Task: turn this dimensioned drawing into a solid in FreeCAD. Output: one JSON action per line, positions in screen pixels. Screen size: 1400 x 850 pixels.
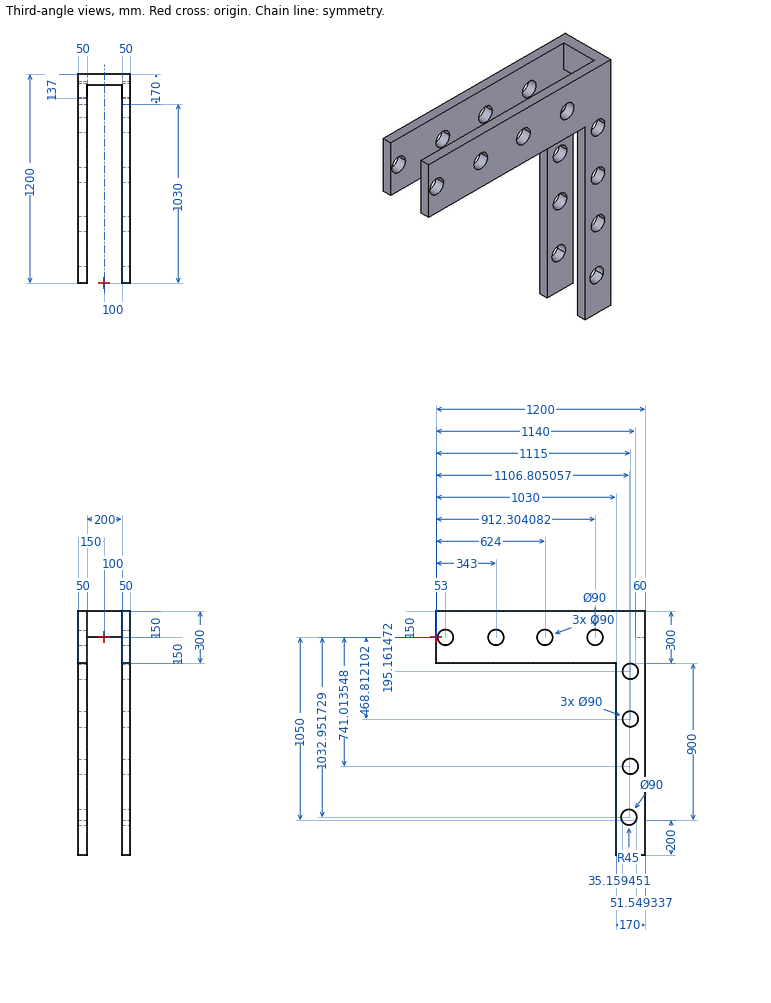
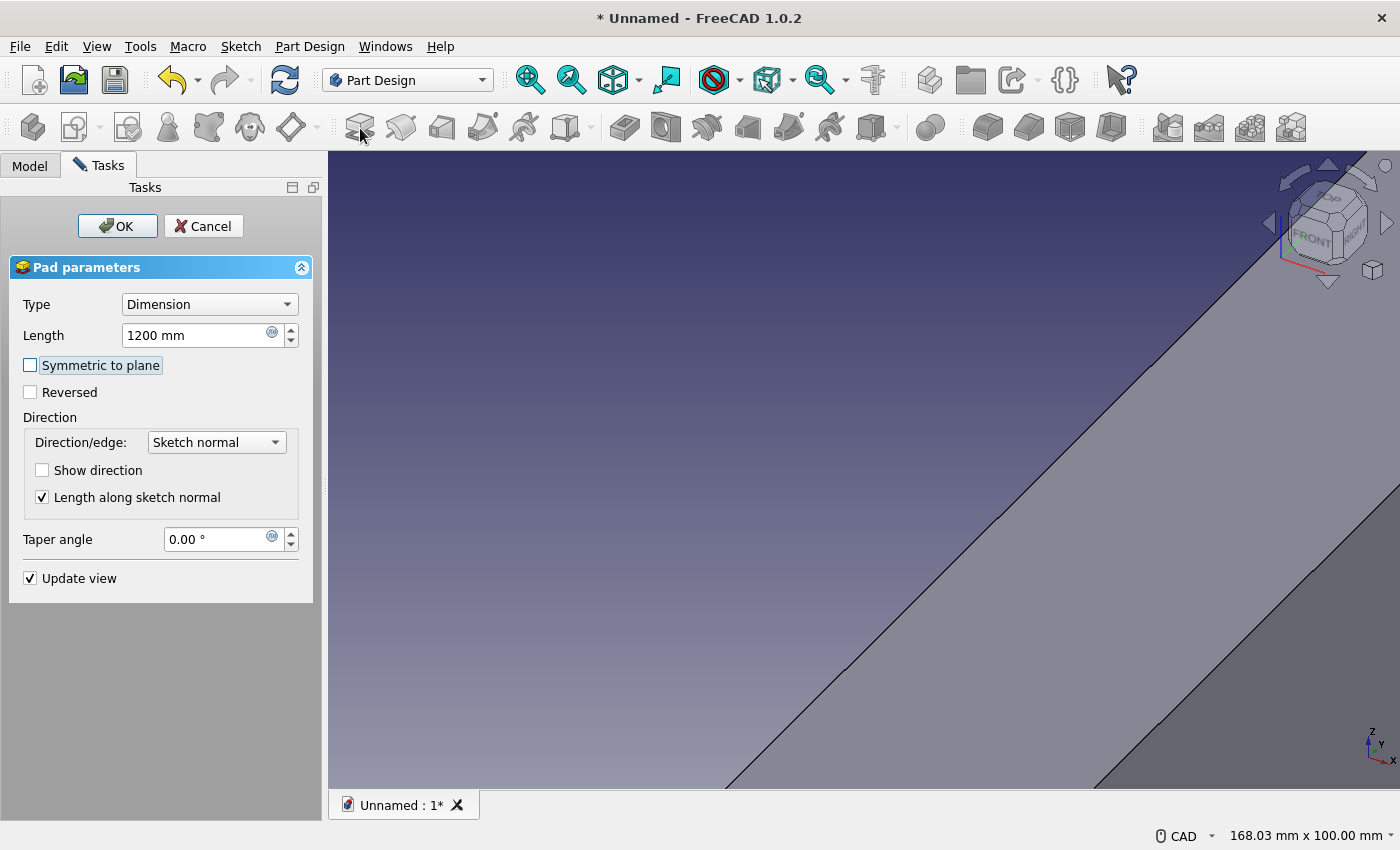
{"action": "left_click", "coordinate": [31, 392]}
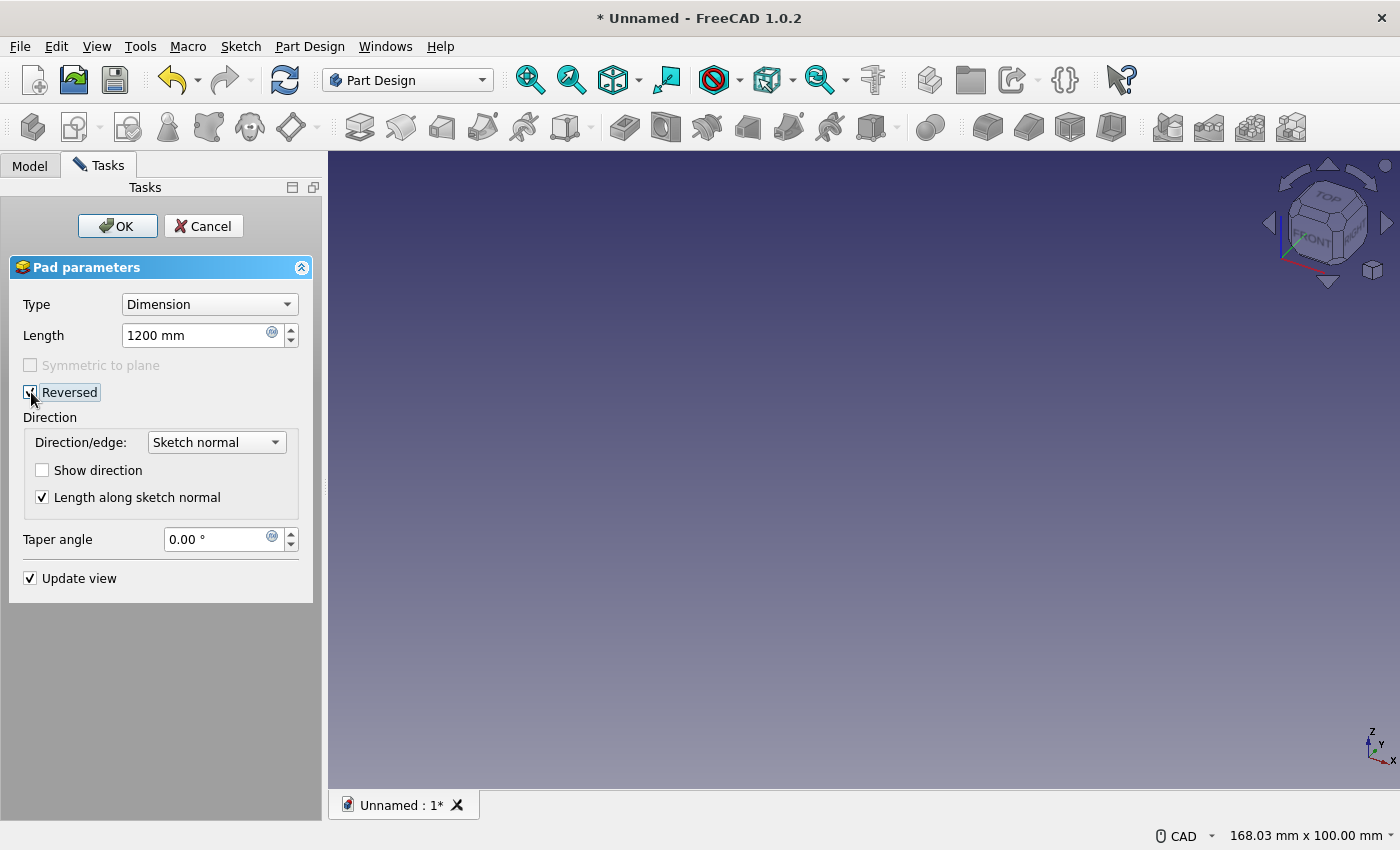
{"action": "left_click", "coordinate": [118, 226]}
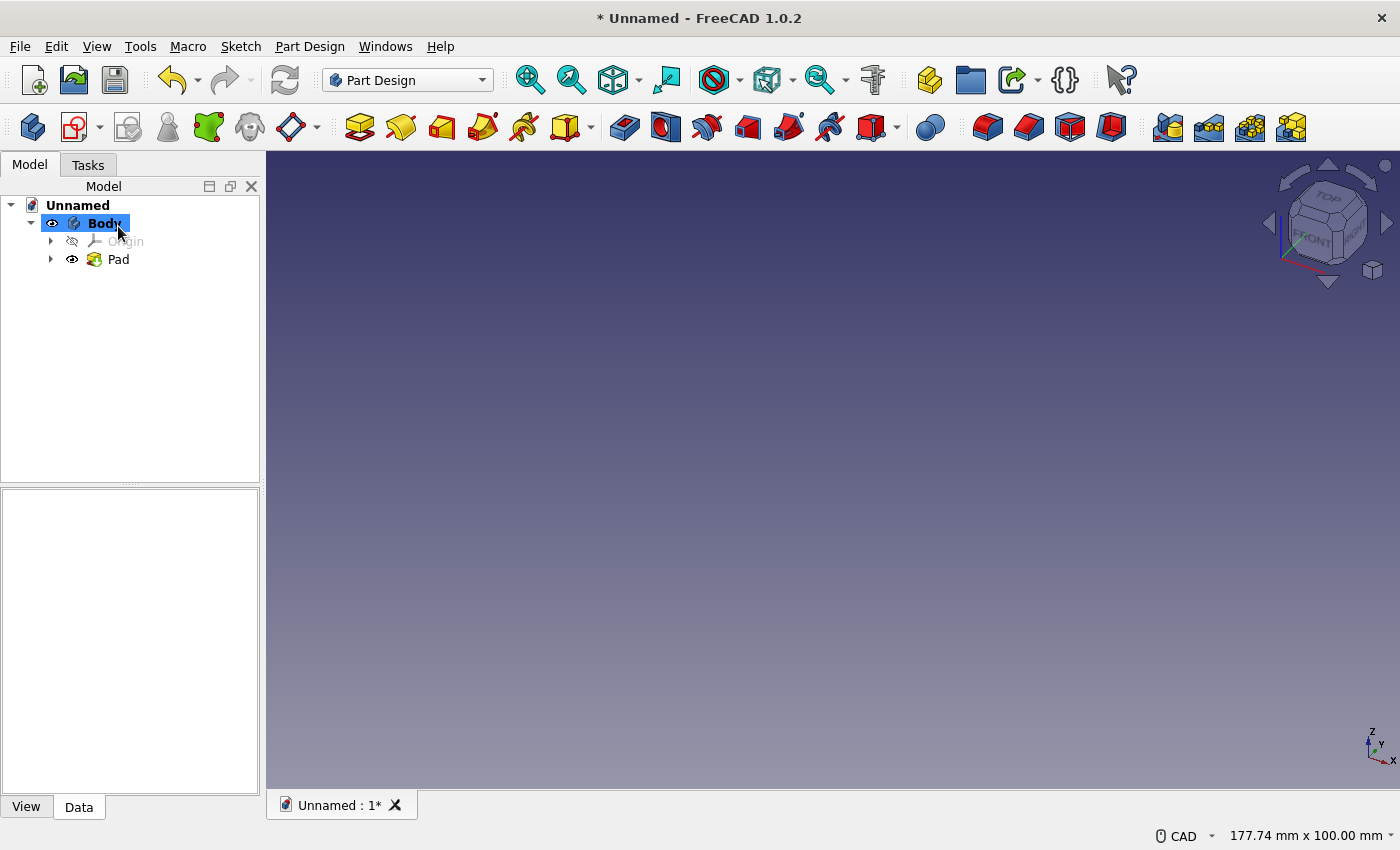
{"action": "left_click", "coordinate": [531, 80]}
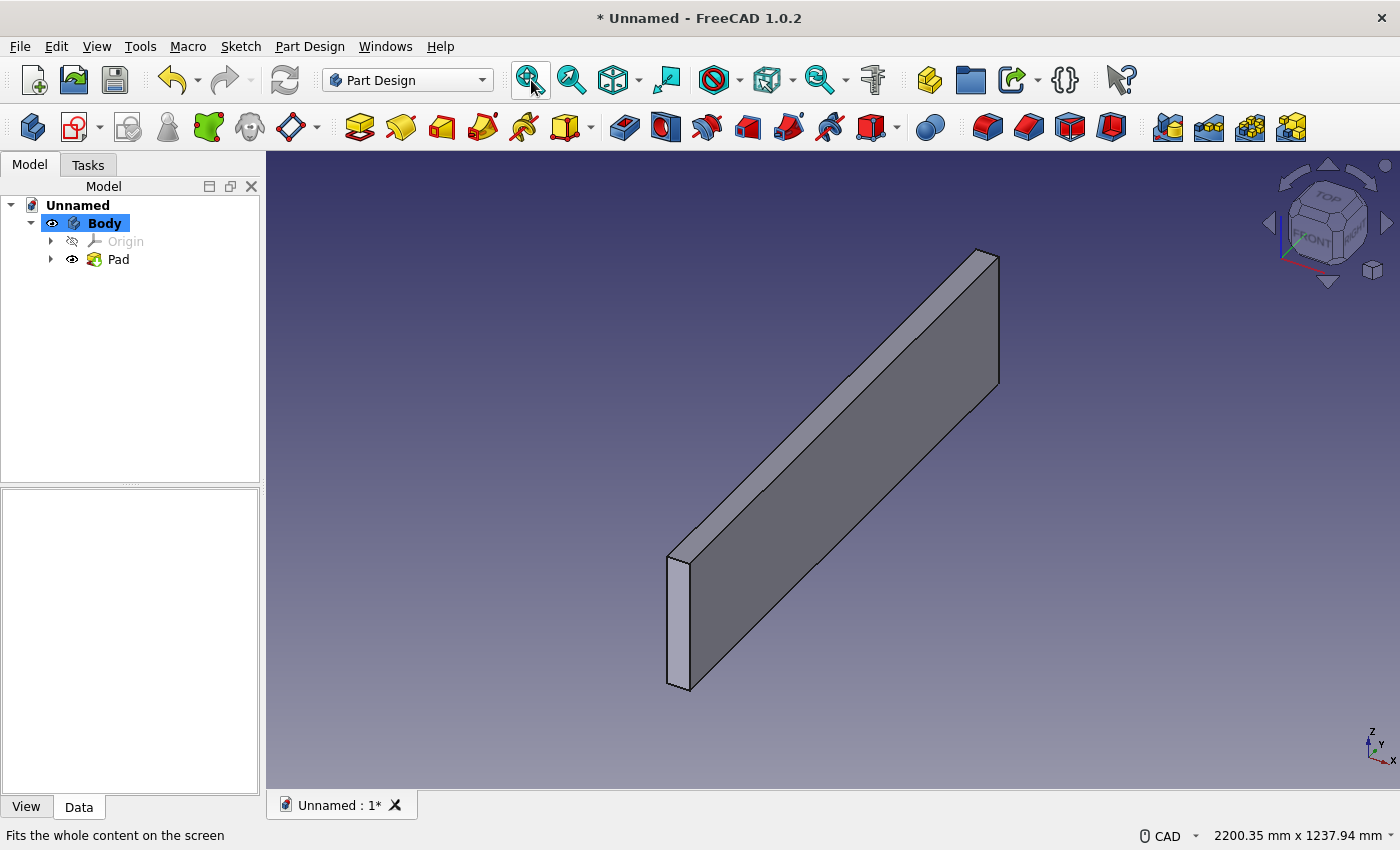
{"action": "left_click", "coordinate": [33, 128]}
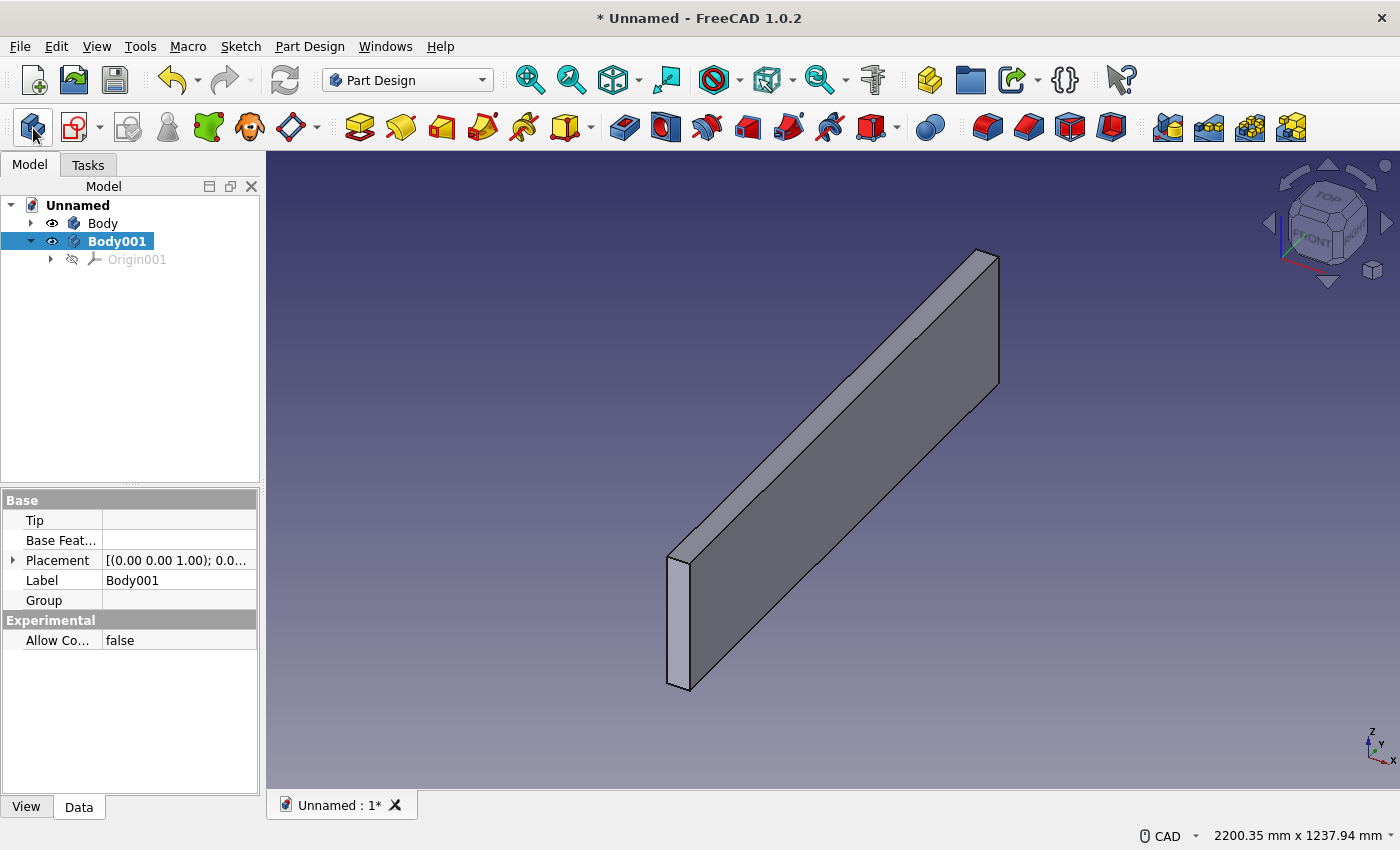
{"action": "left_click", "coordinate": [306, 749]}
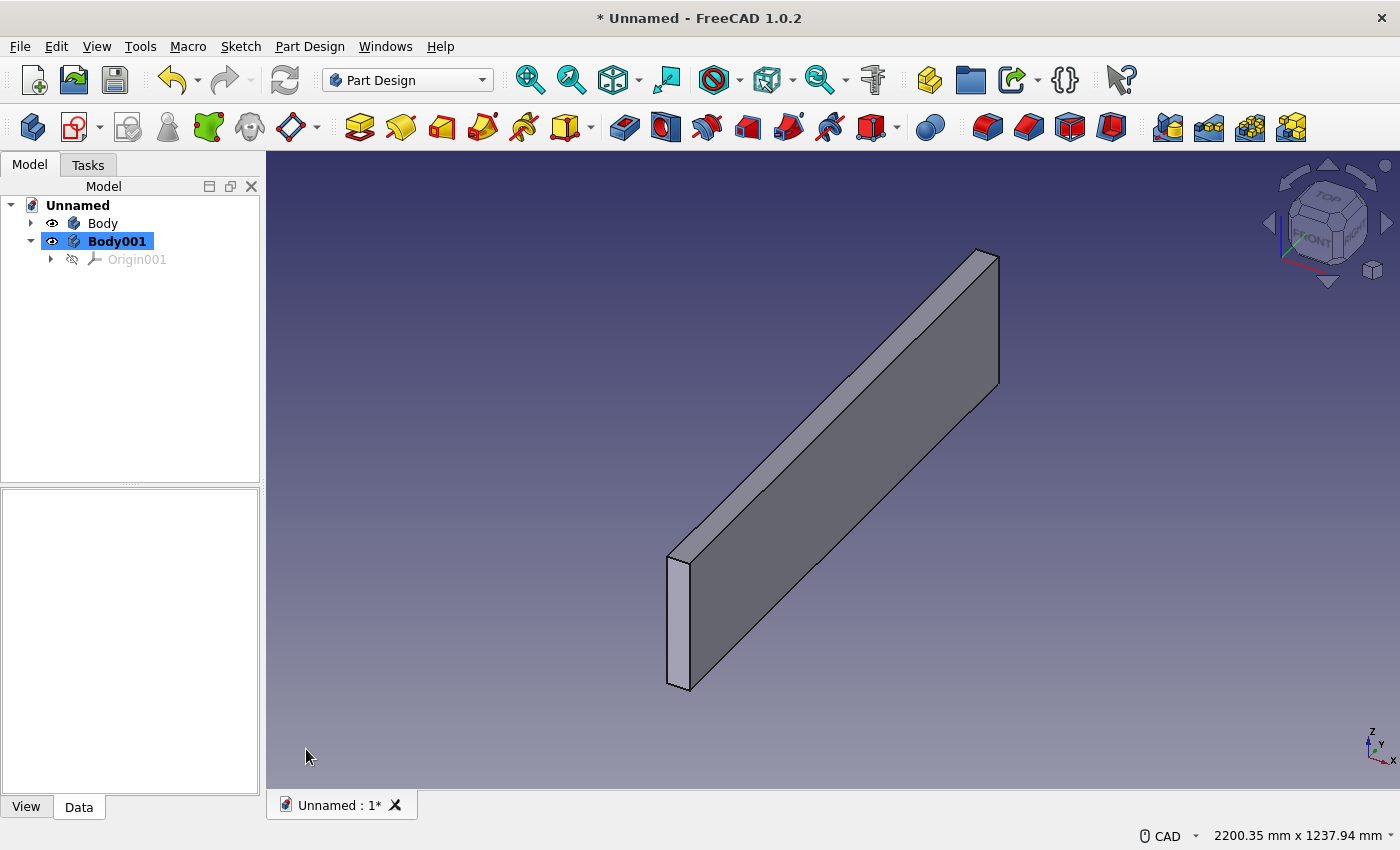
{"action": "left_click", "coordinate": [74, 128]}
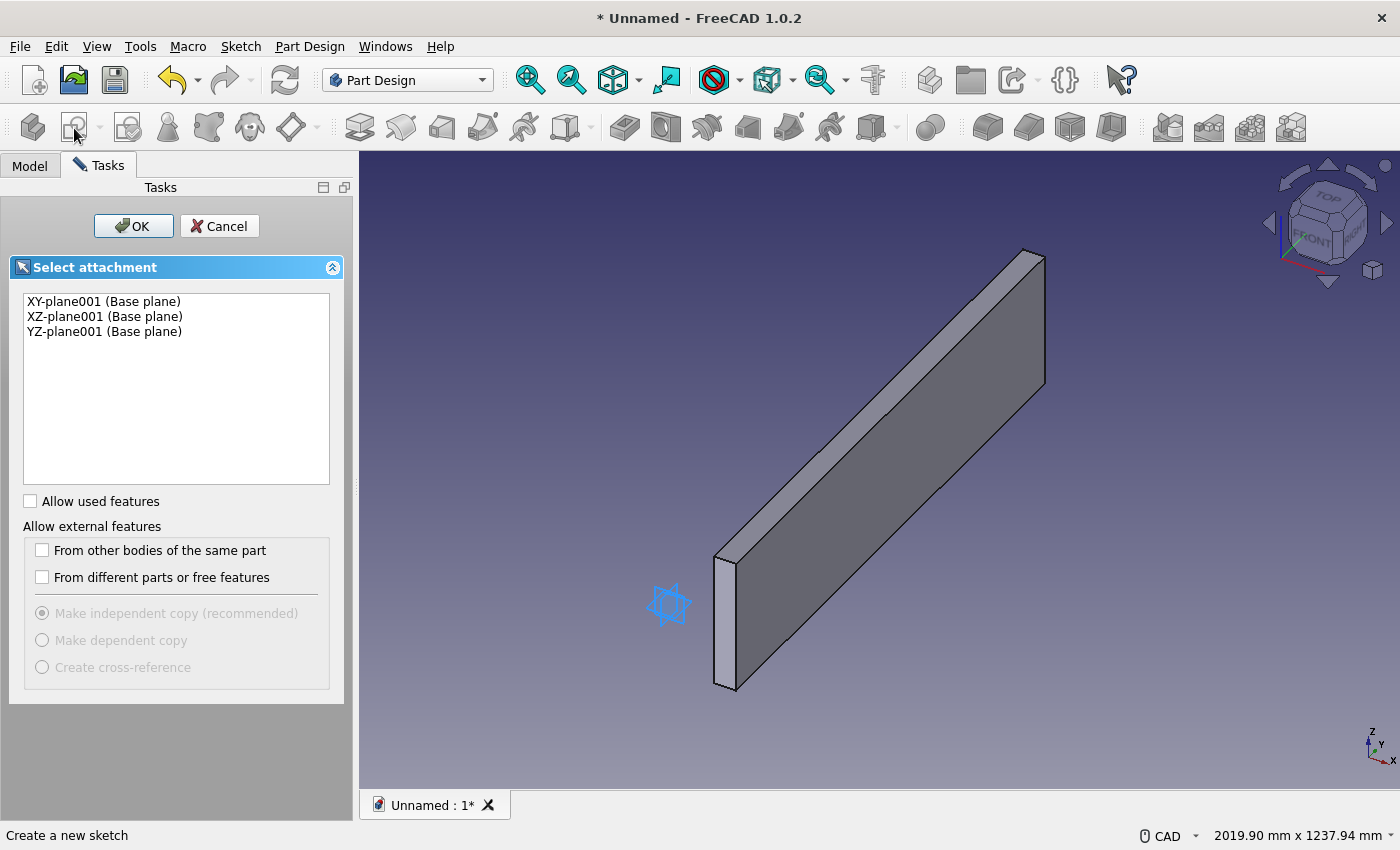
{"action": "left_click", "coordinate": [84, 316]}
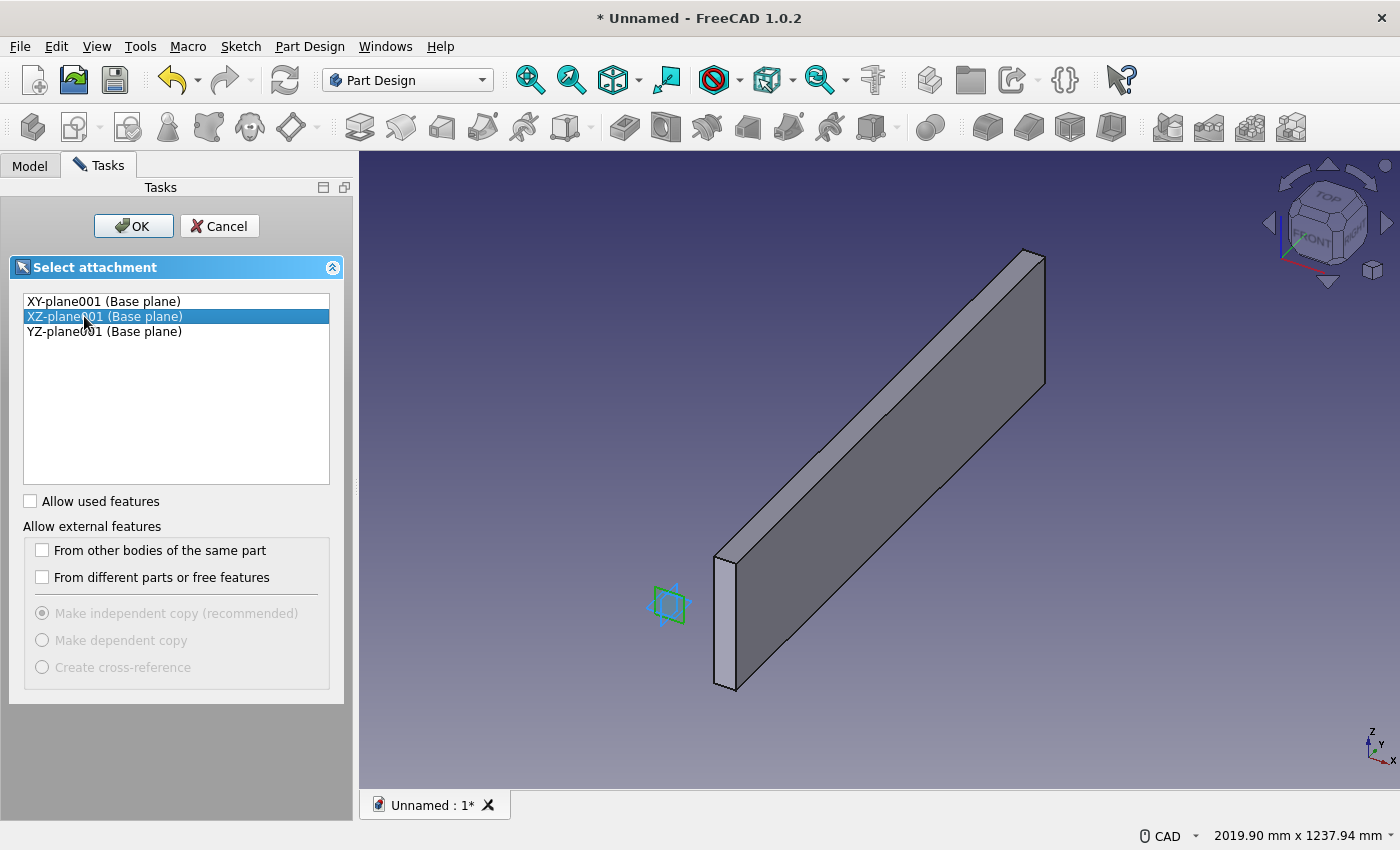
{"action": "left_click", "coordinate": [134, 226]}